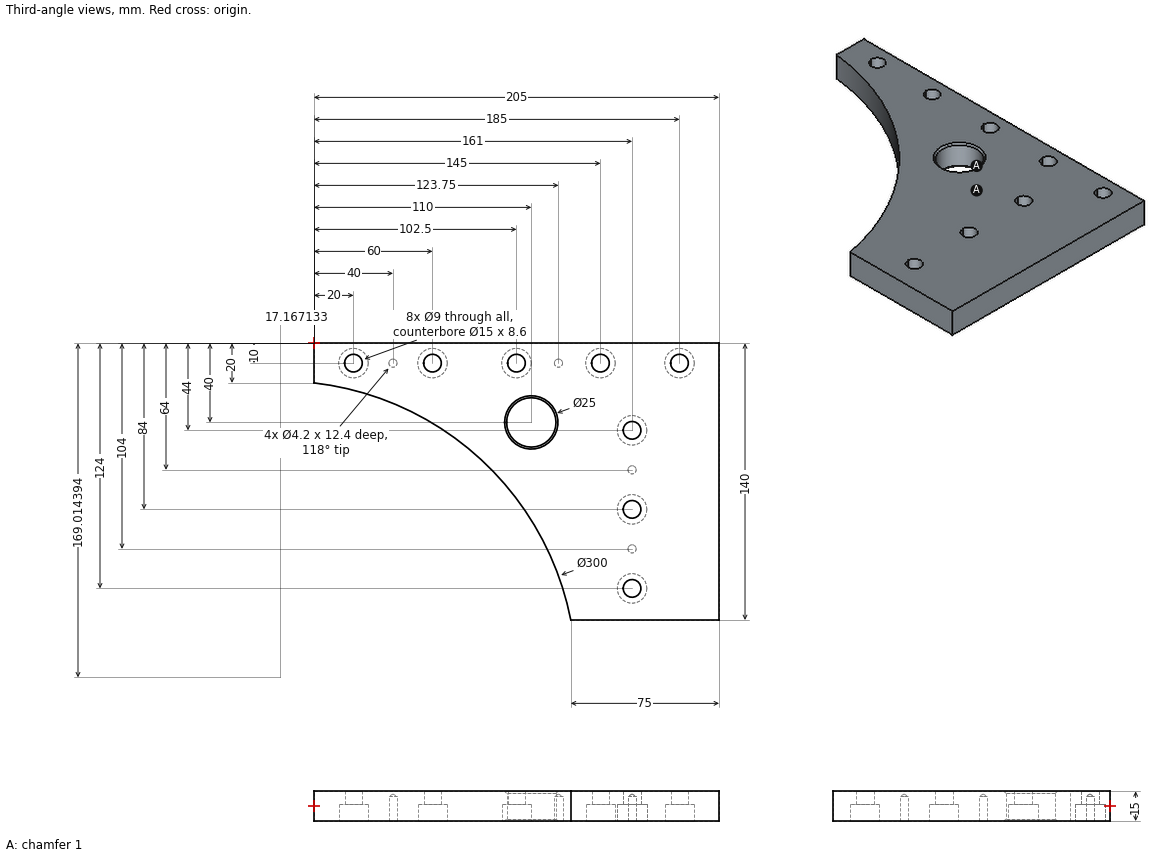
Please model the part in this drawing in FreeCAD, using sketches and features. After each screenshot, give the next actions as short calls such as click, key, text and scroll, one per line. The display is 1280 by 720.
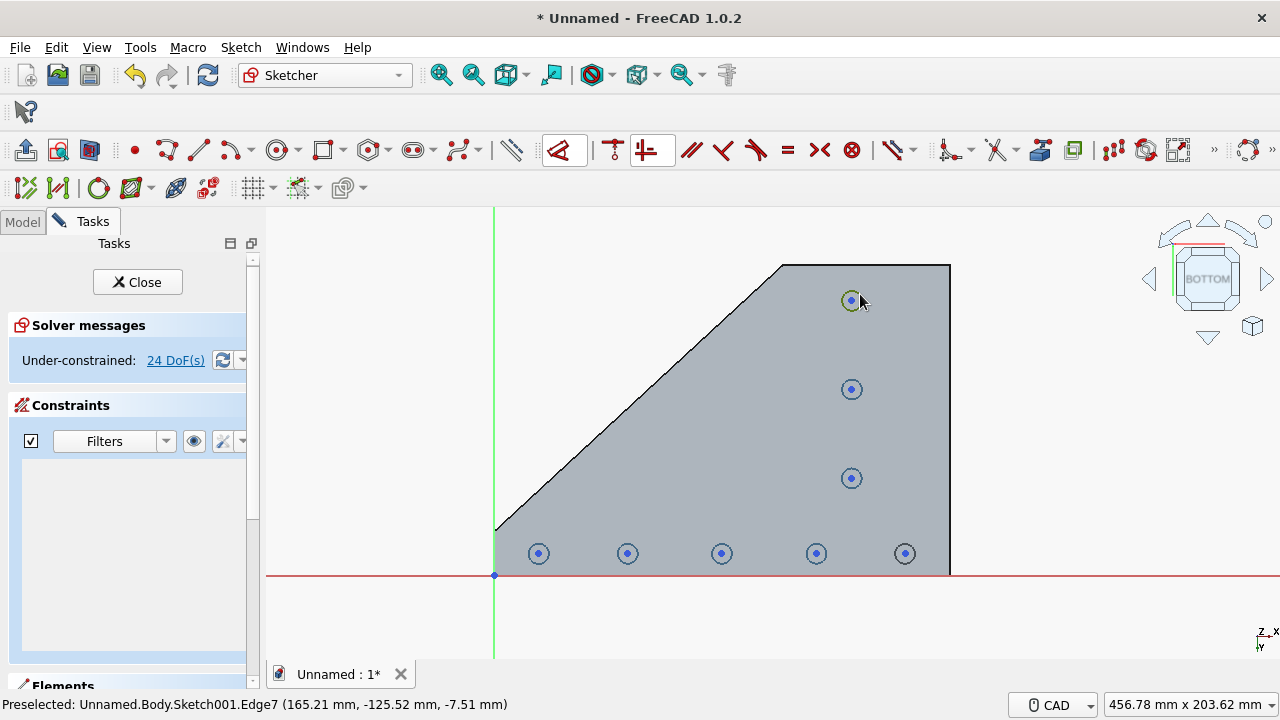
scroll(912, 547, up, 2)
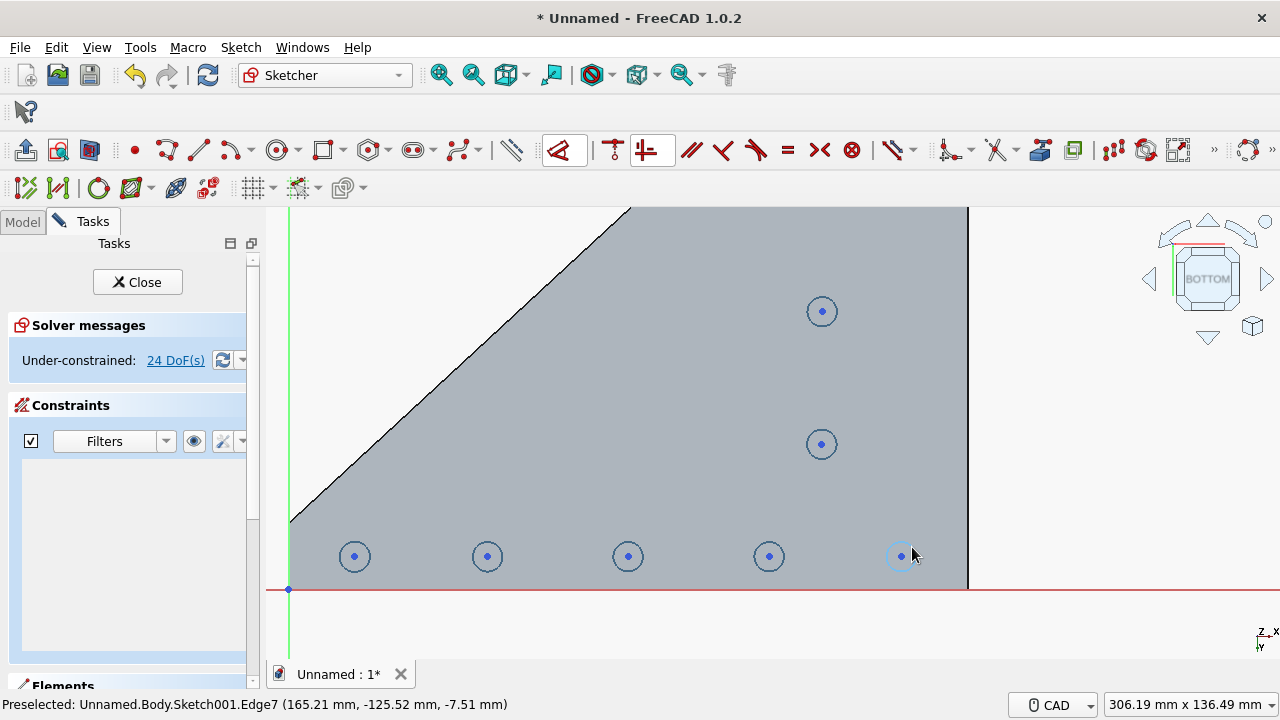
click(912, 546)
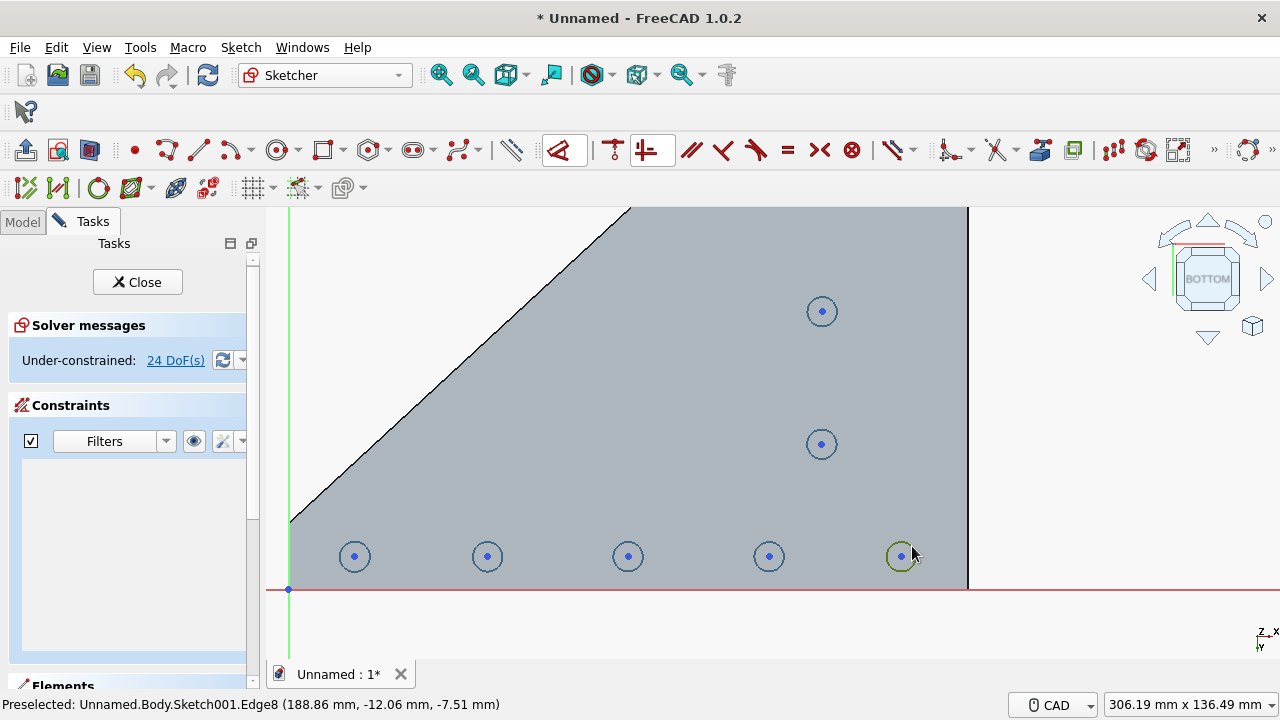
click(788, 150)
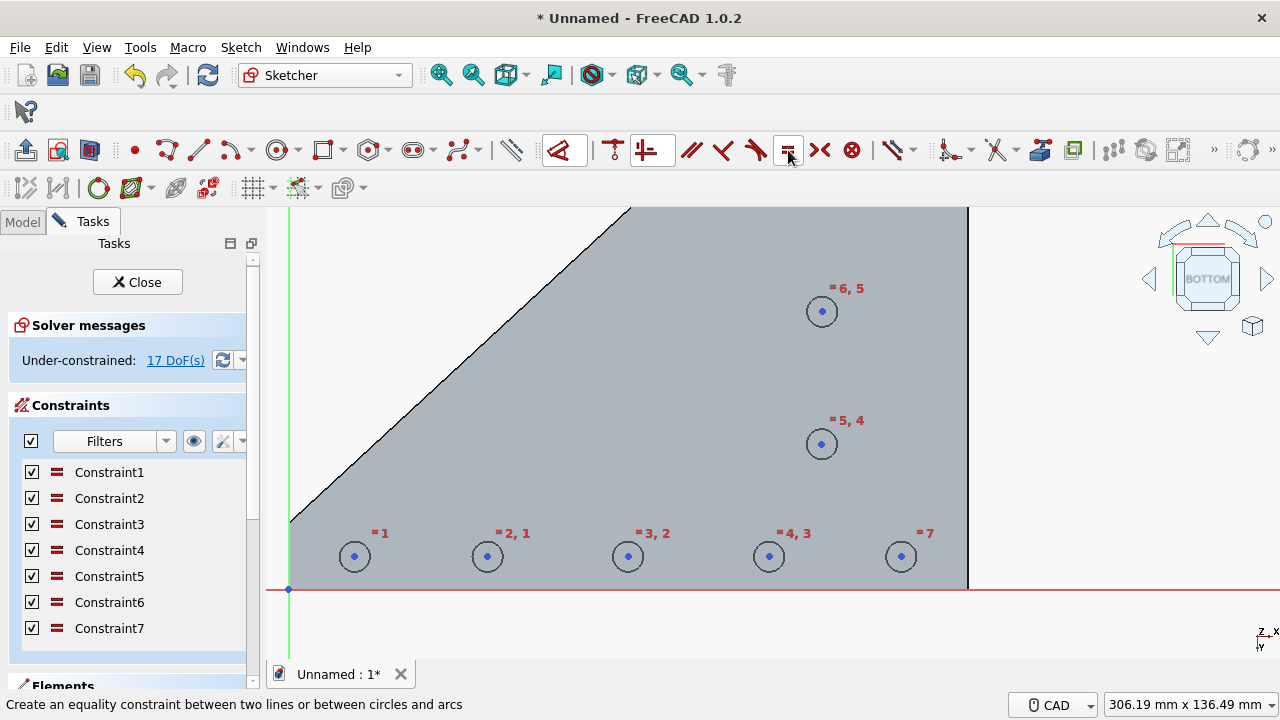
scroll(365, 546, up, 2)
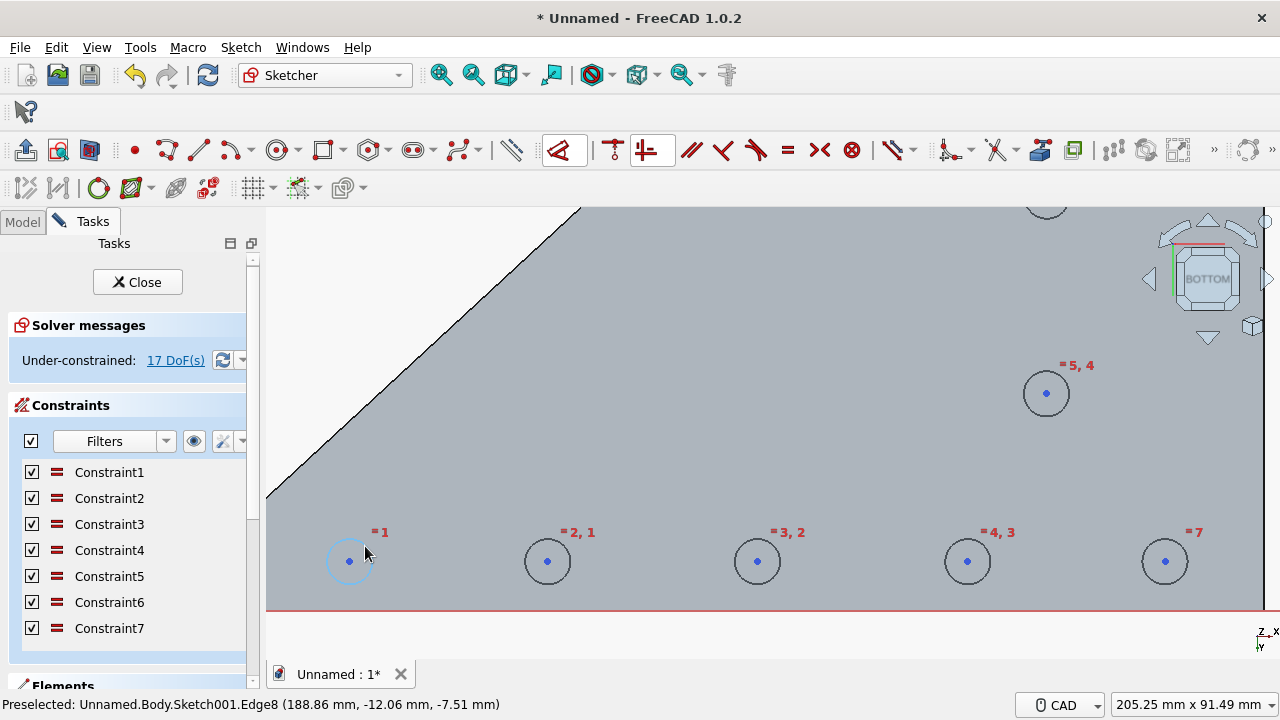
click(366, 546)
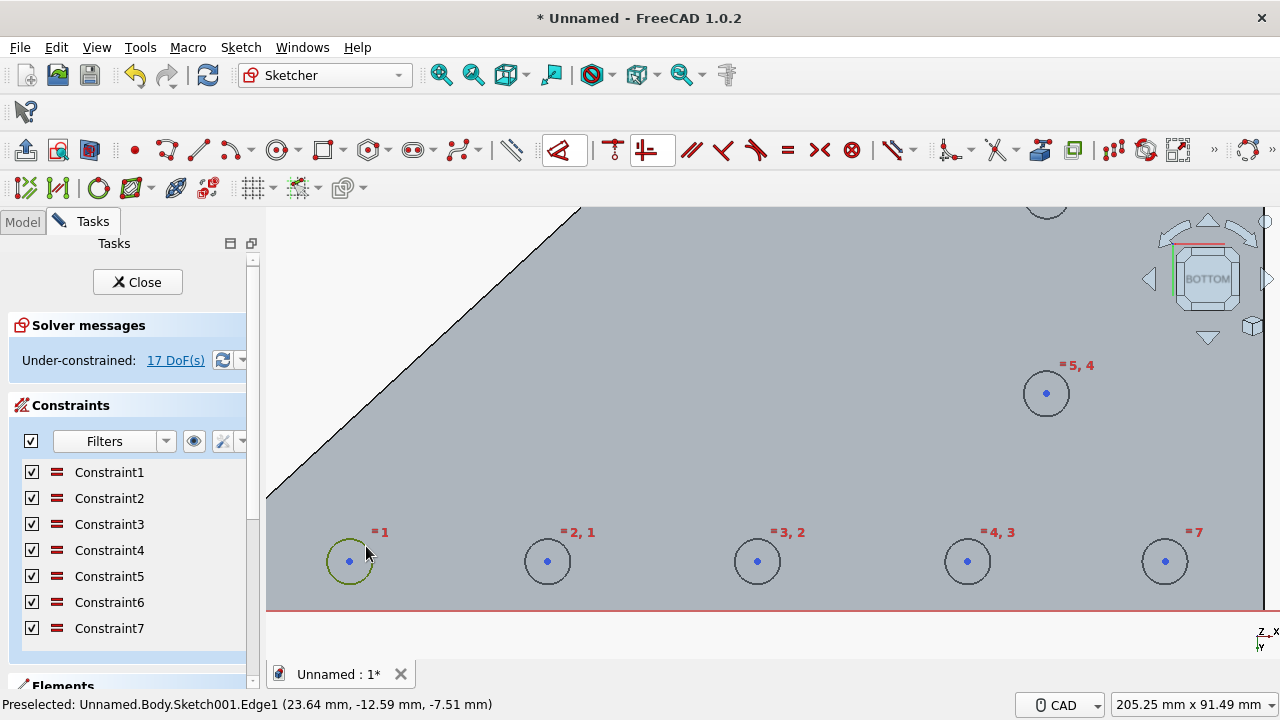
key(k)
key(o)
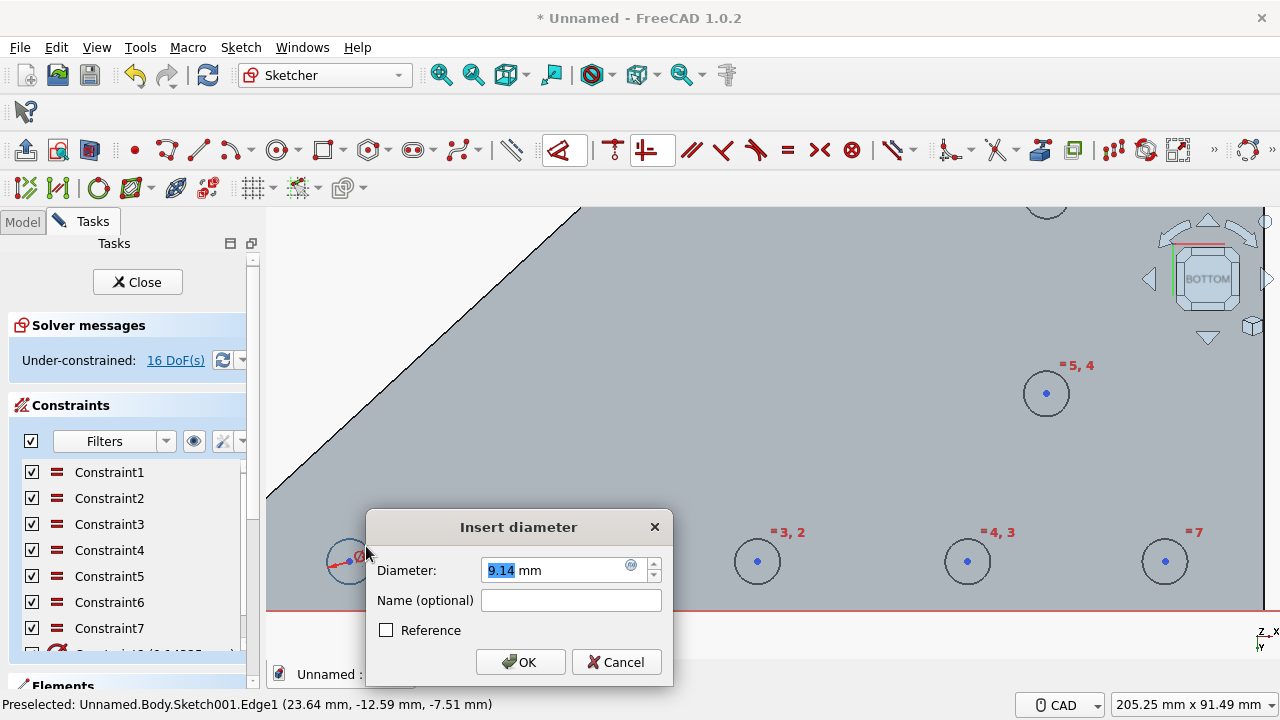
text(9)
key(Return)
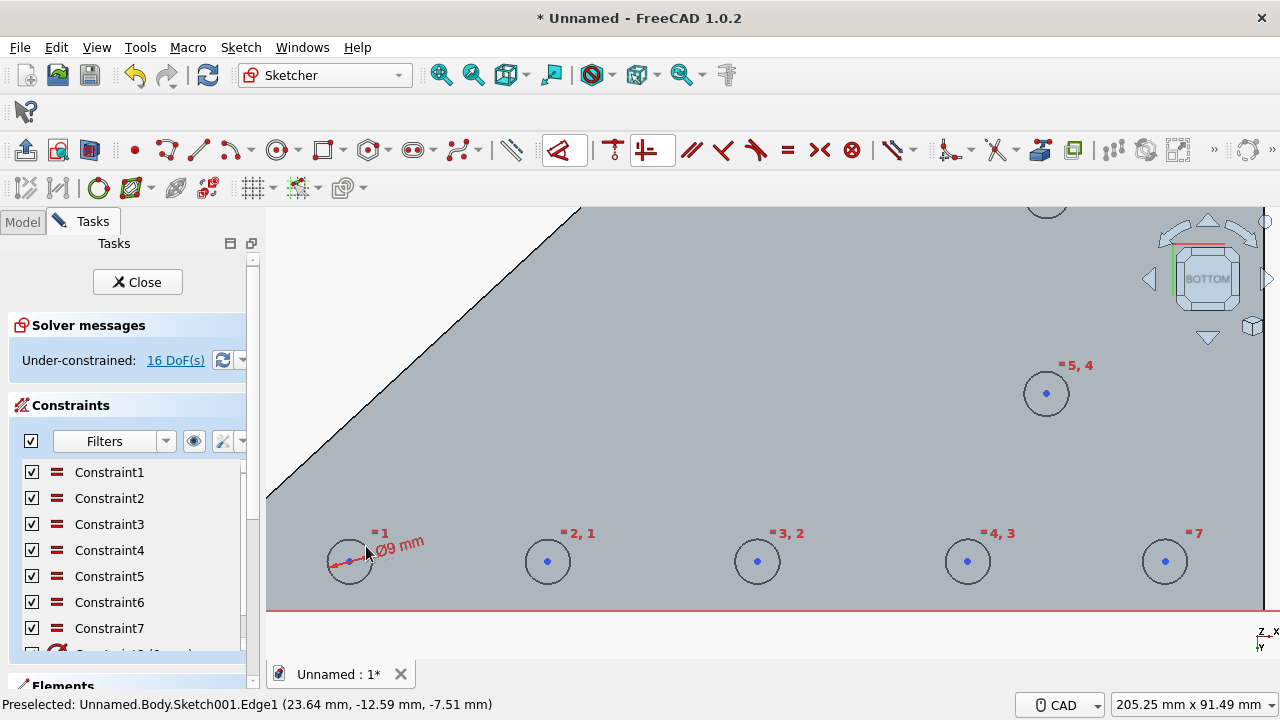
click(350, 562)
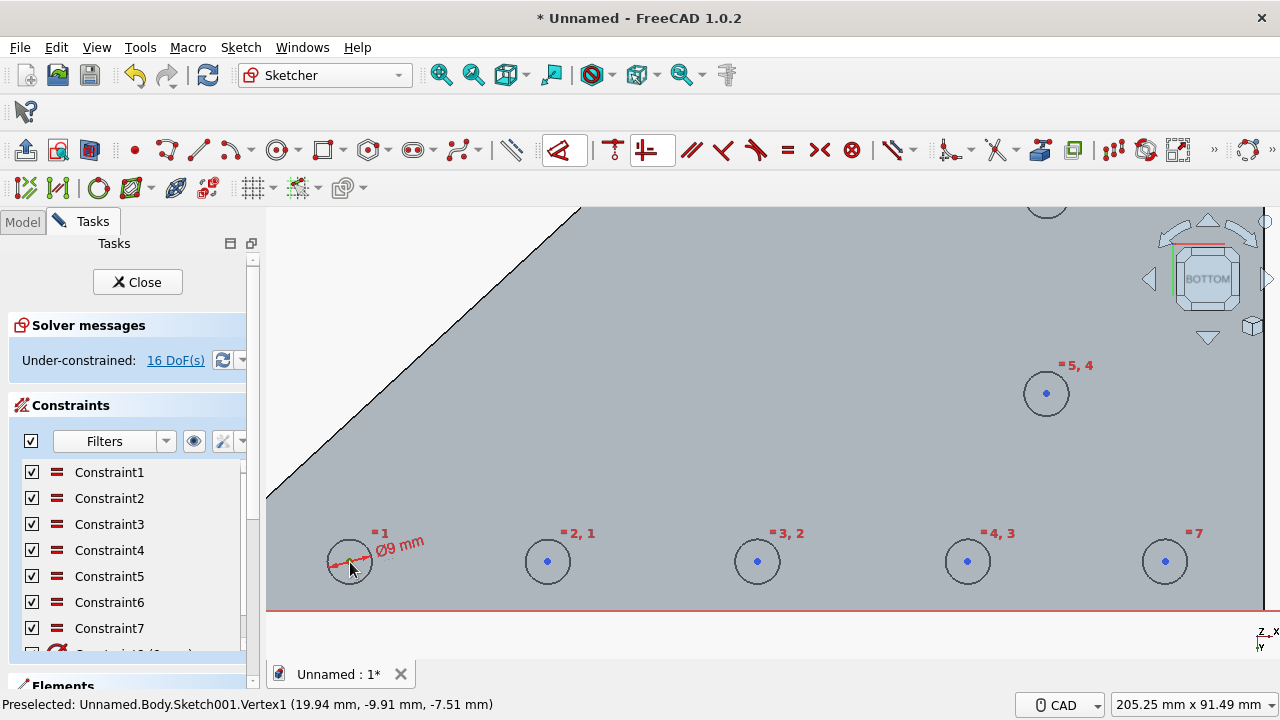
click(582, 150)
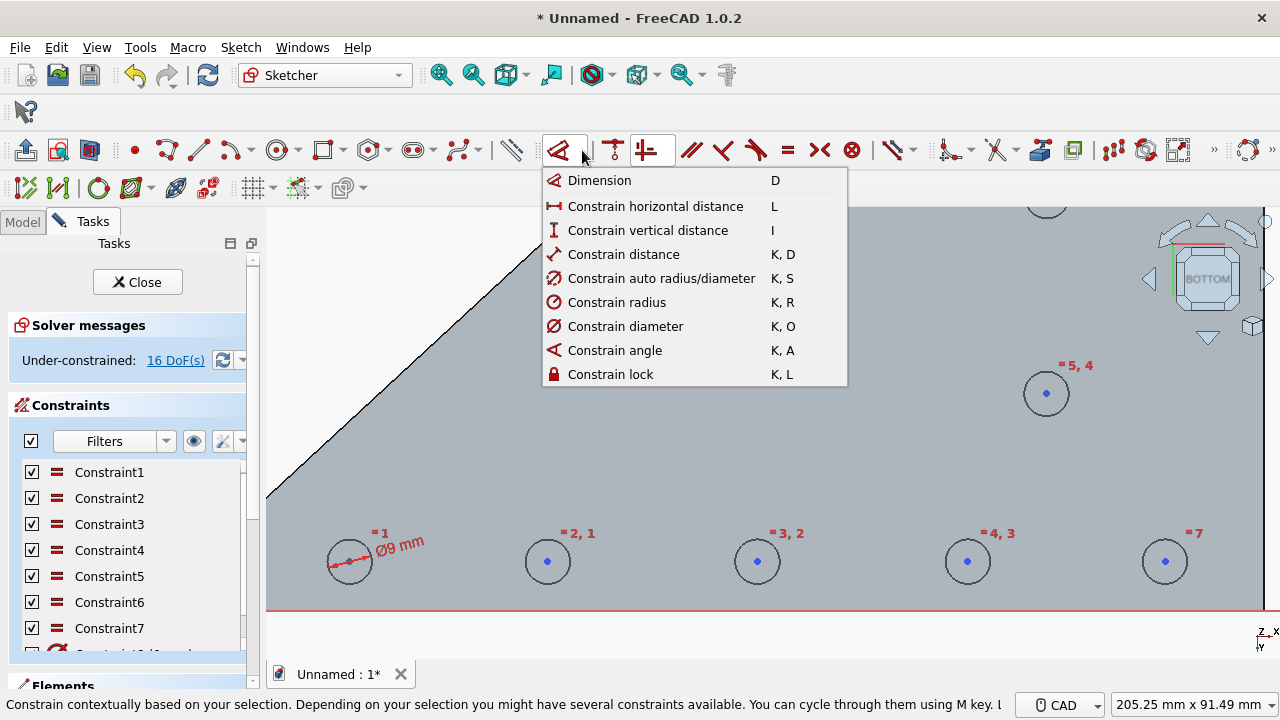
click(695, 206)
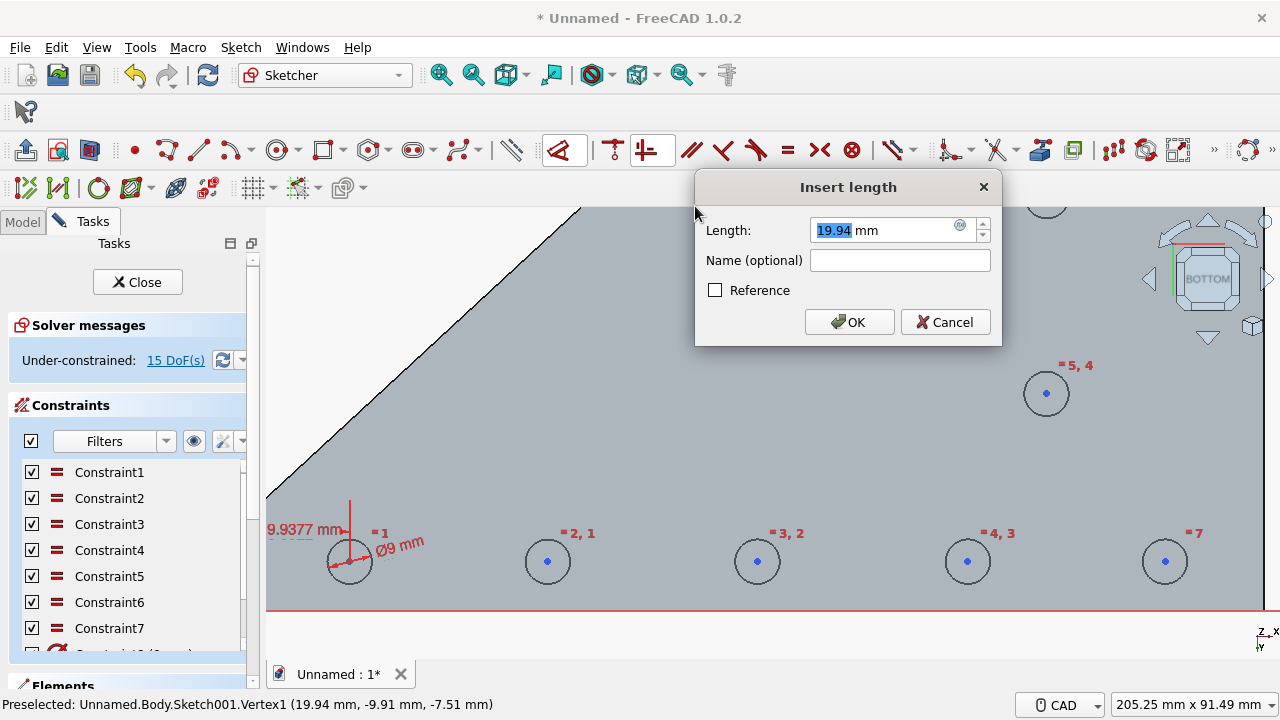
text(20)
key(Return)